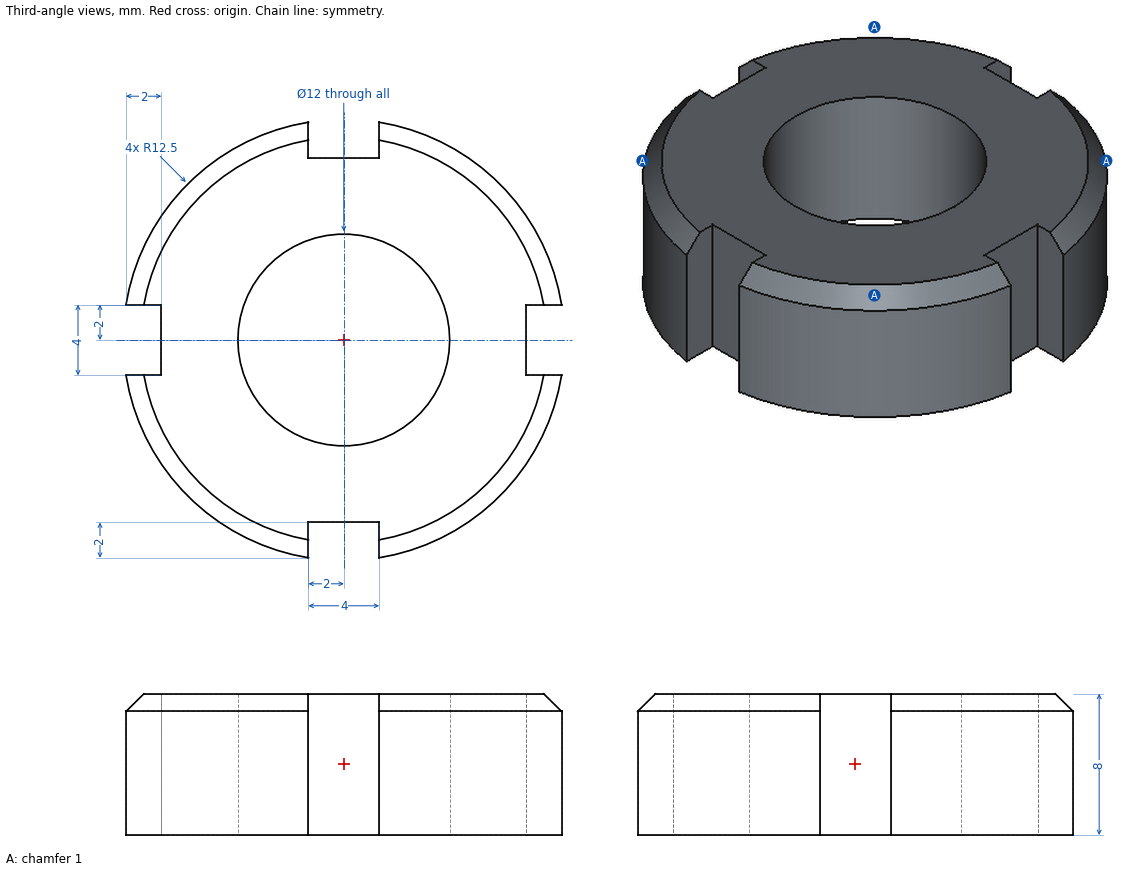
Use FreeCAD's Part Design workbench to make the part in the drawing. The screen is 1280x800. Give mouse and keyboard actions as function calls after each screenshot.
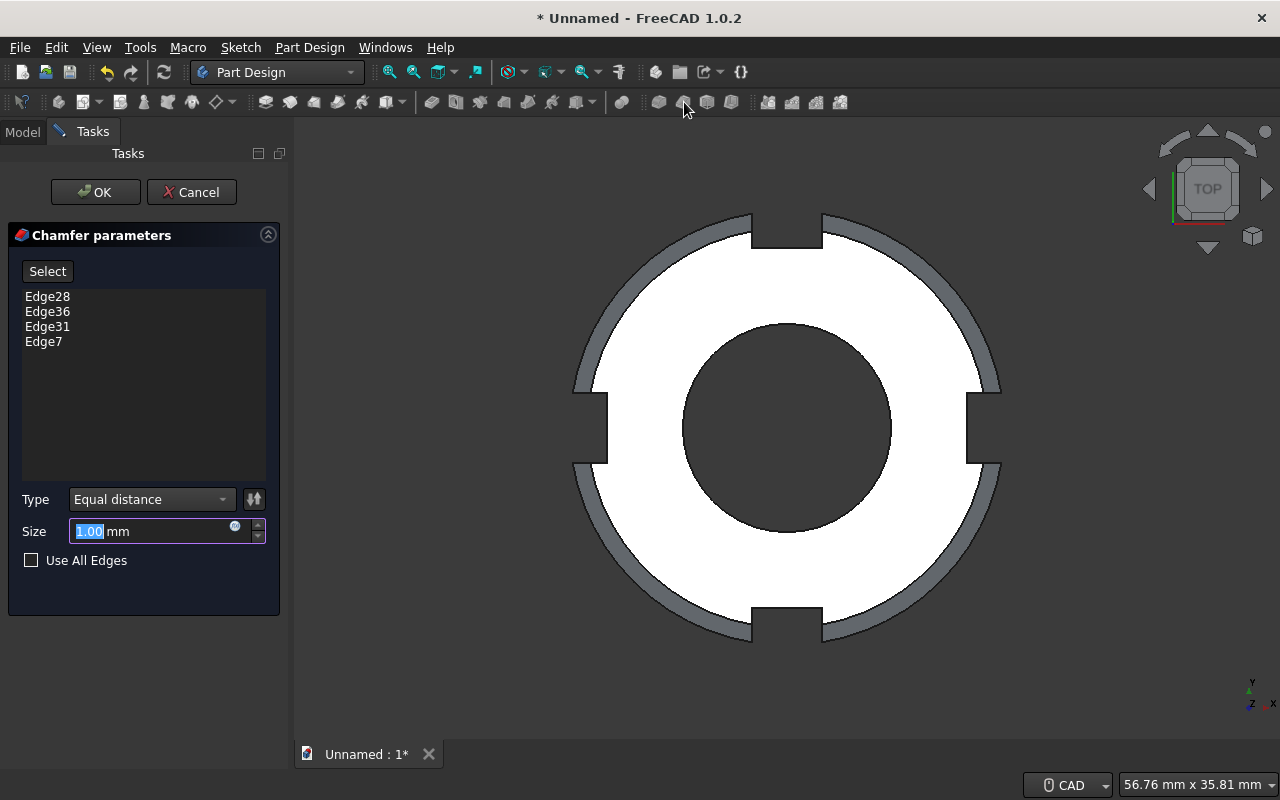
text(1)
key(Tab)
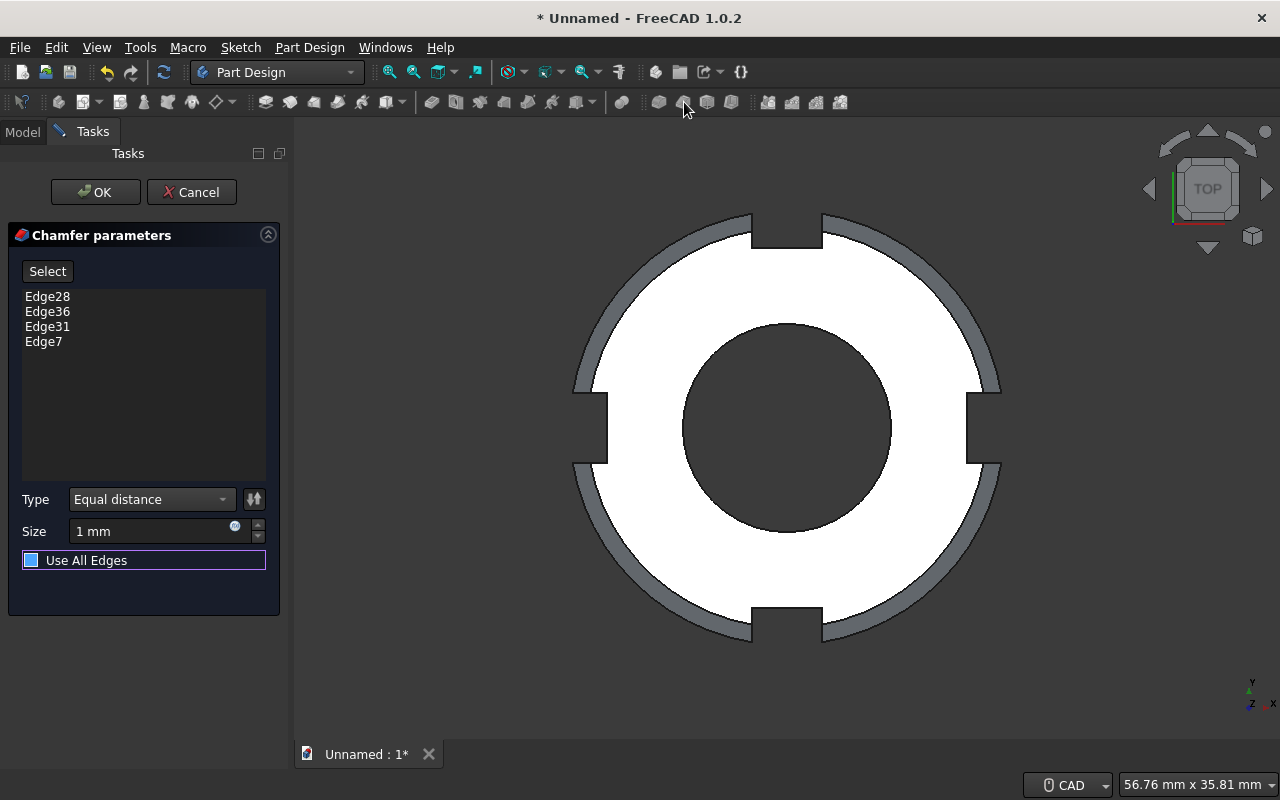
click(96, 192)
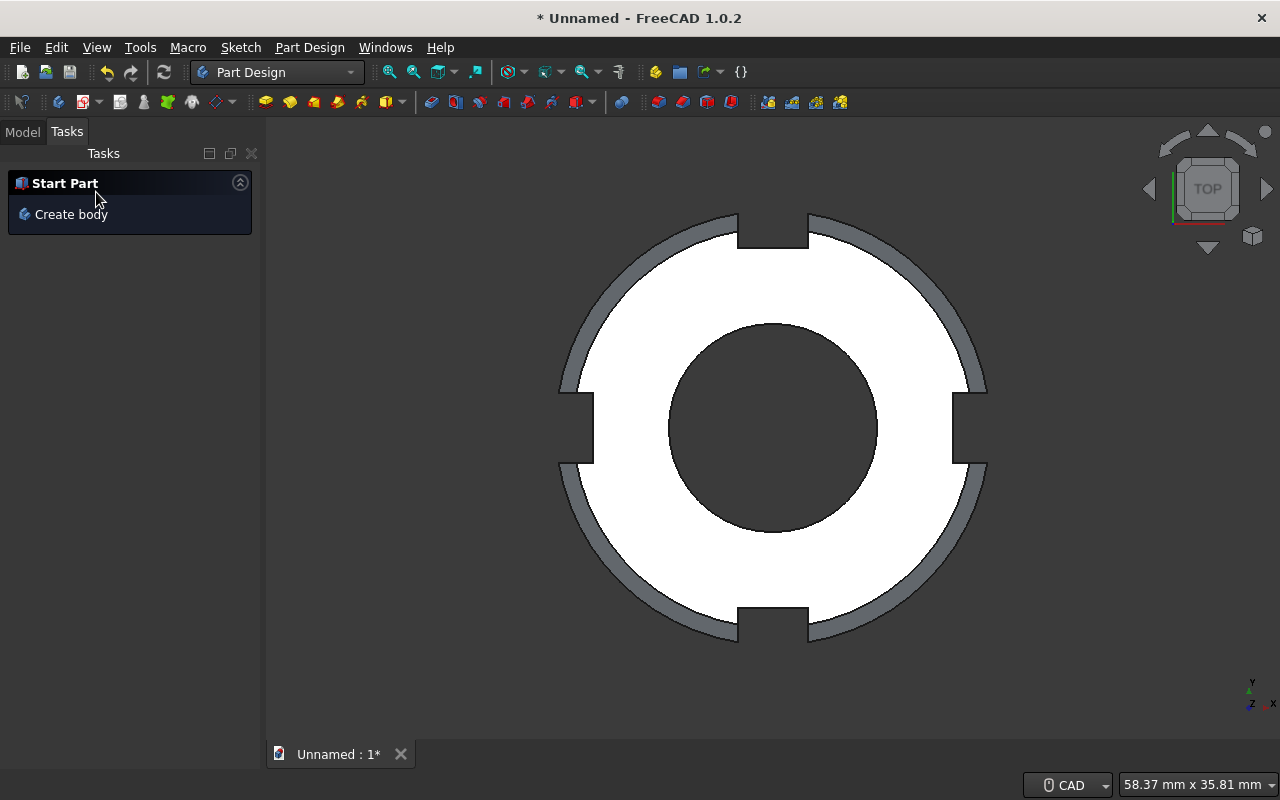
key(0)